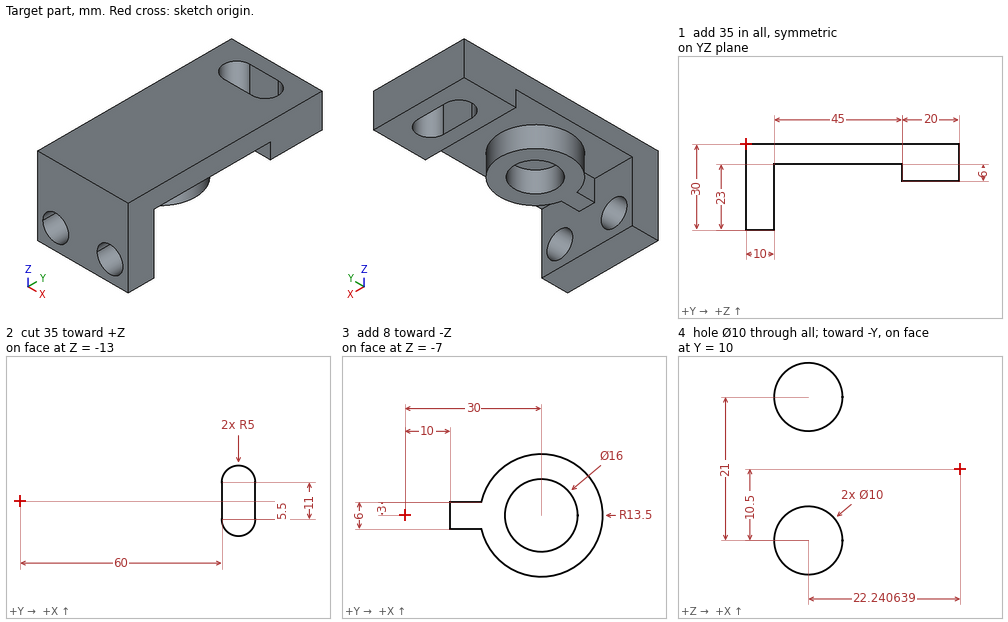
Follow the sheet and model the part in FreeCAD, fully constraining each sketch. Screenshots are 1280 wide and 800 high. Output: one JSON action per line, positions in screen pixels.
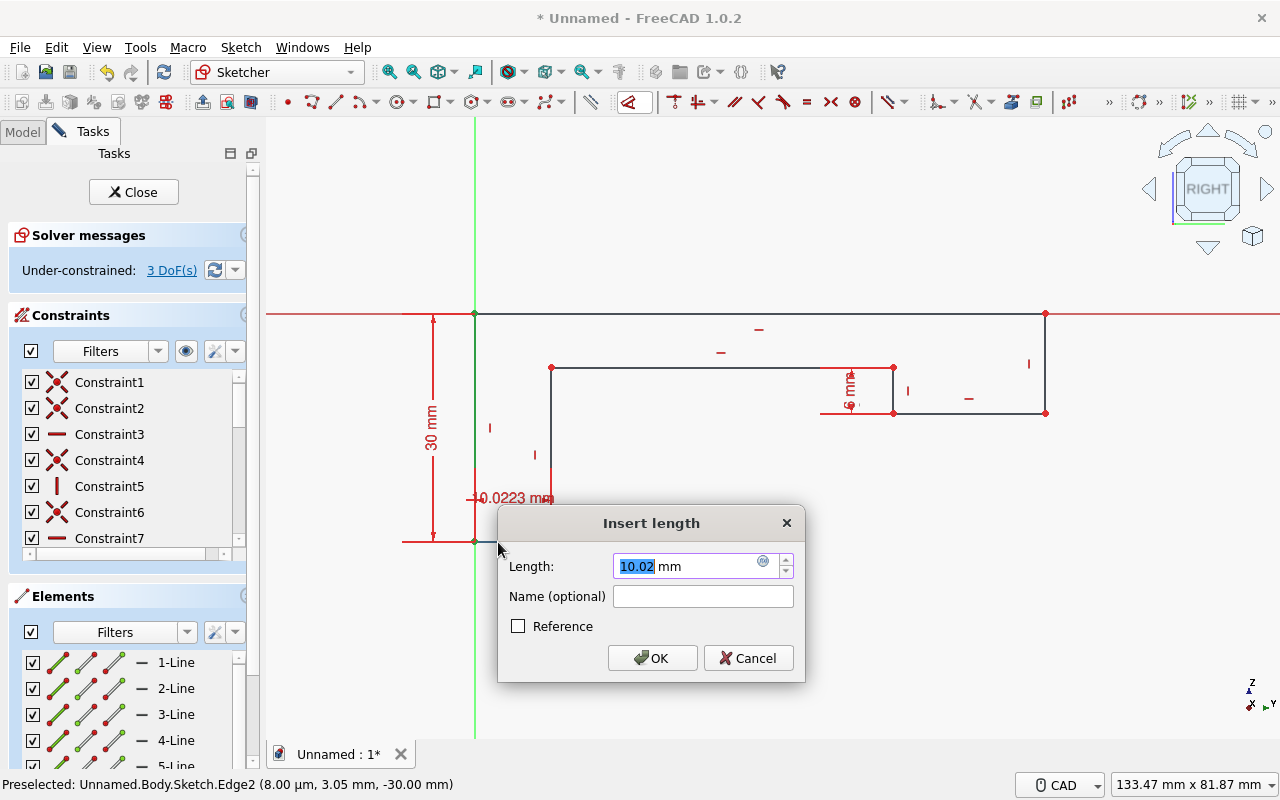
{"action": "type", "text": "10"}
{"action": "key", "text": "Return"}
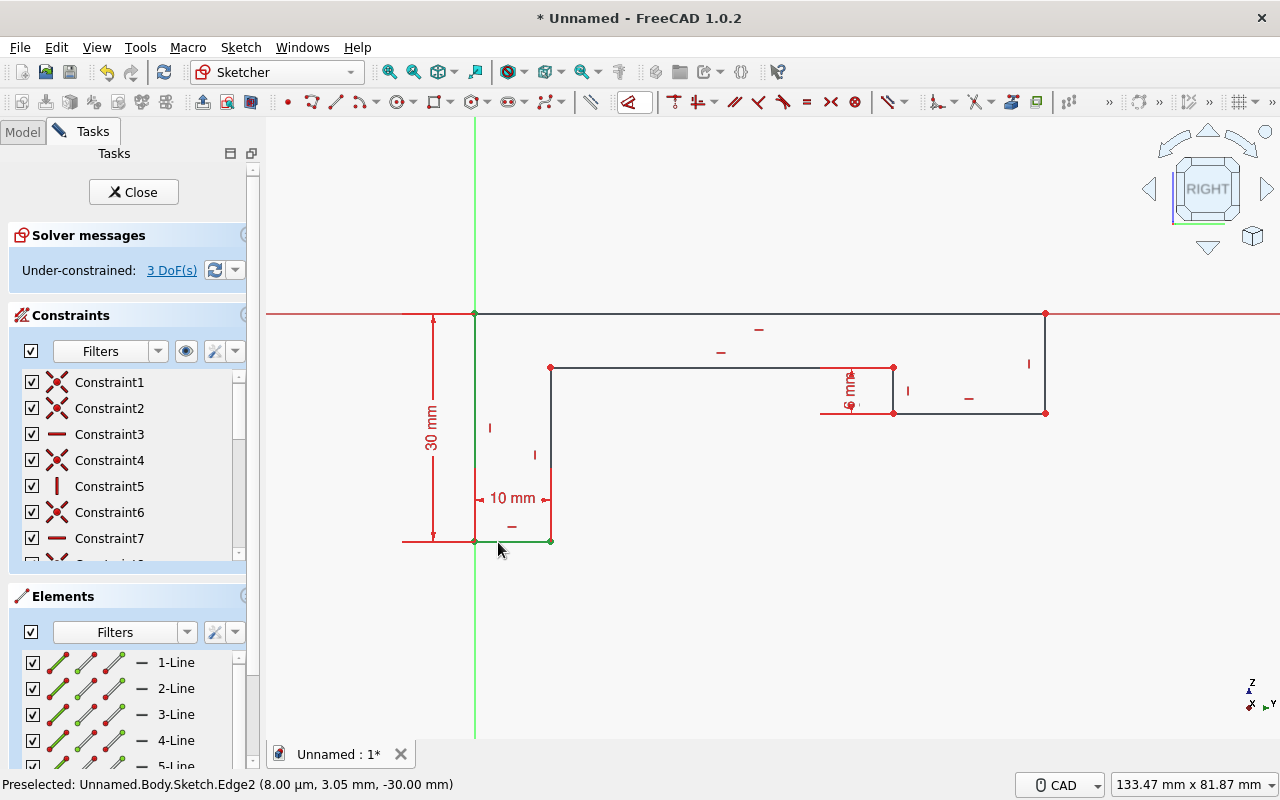
{"action": "left_click", "coordinate": [551, 490]}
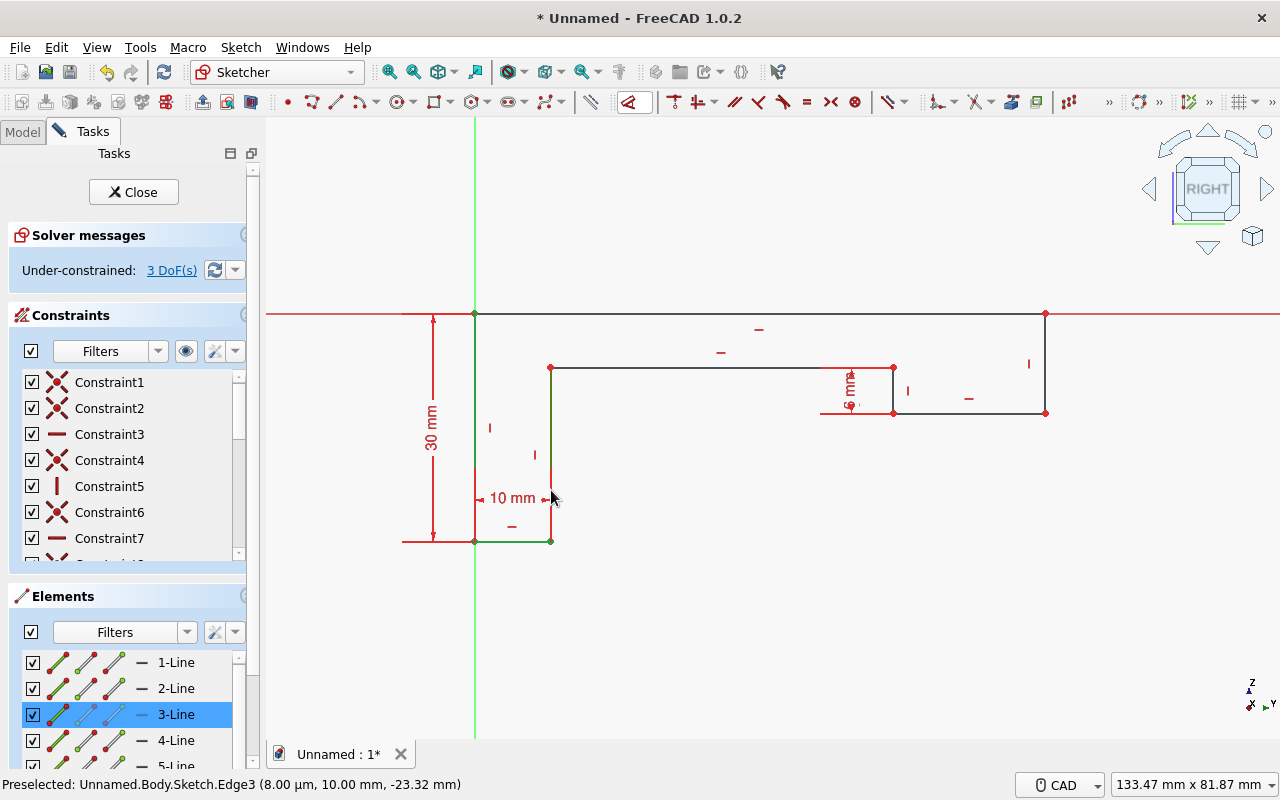
{"action": "key", "text": "i"}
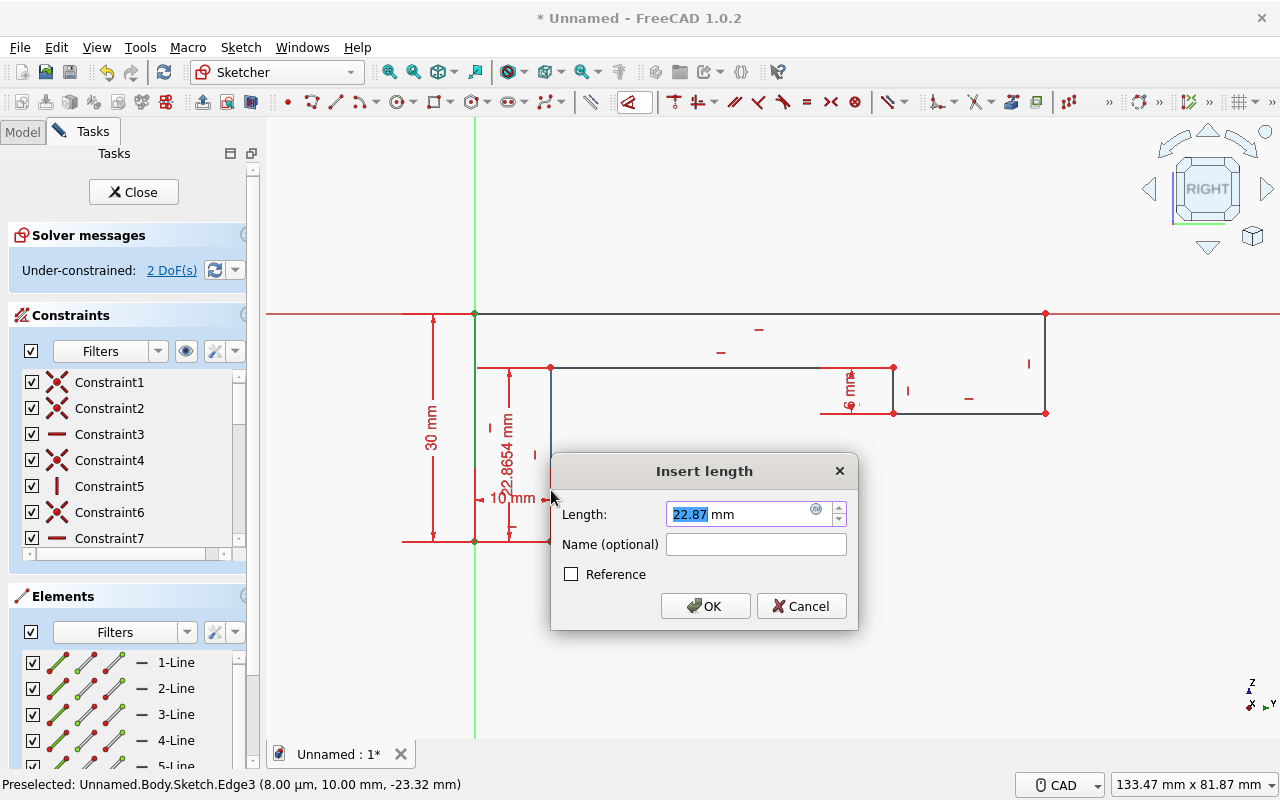
{"action": "type", "text": "23"}
{"action": "key", "text": "Return"}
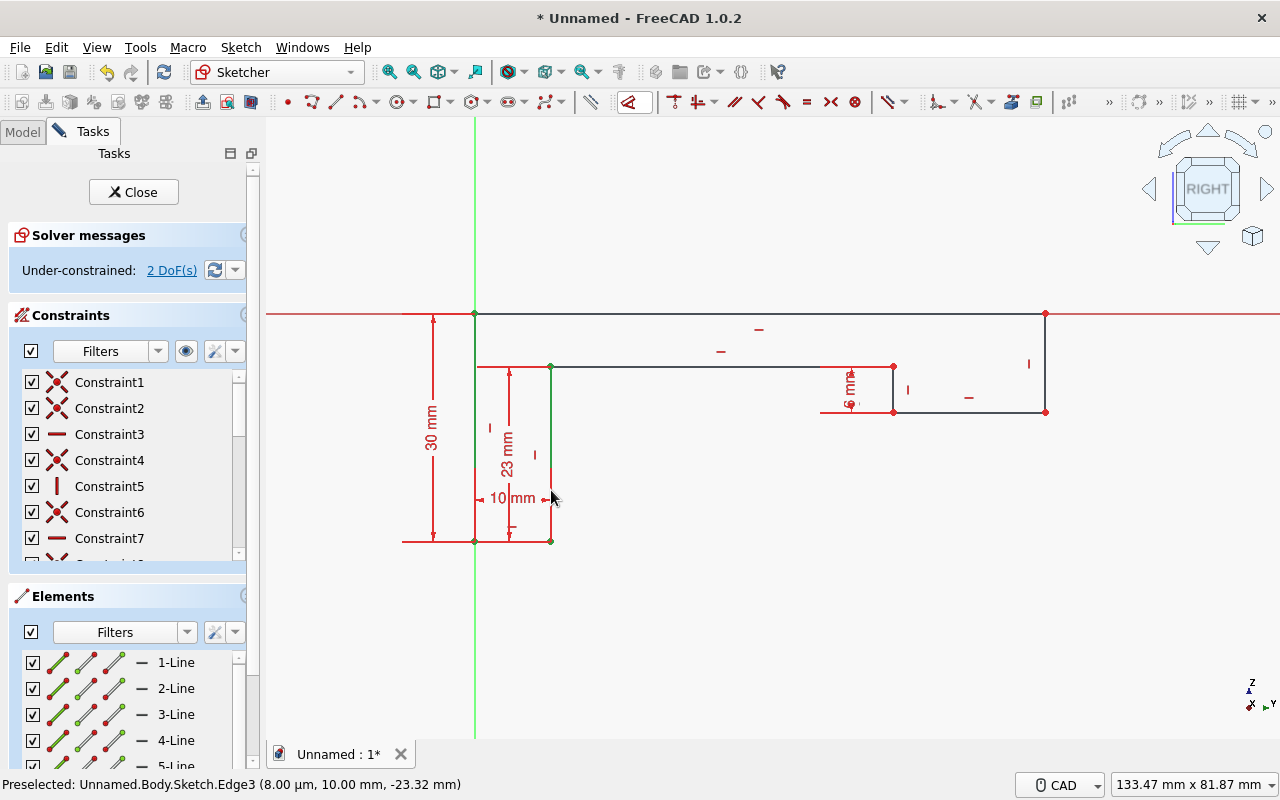
{"action": "left_click", "coordinate": [653, 367]}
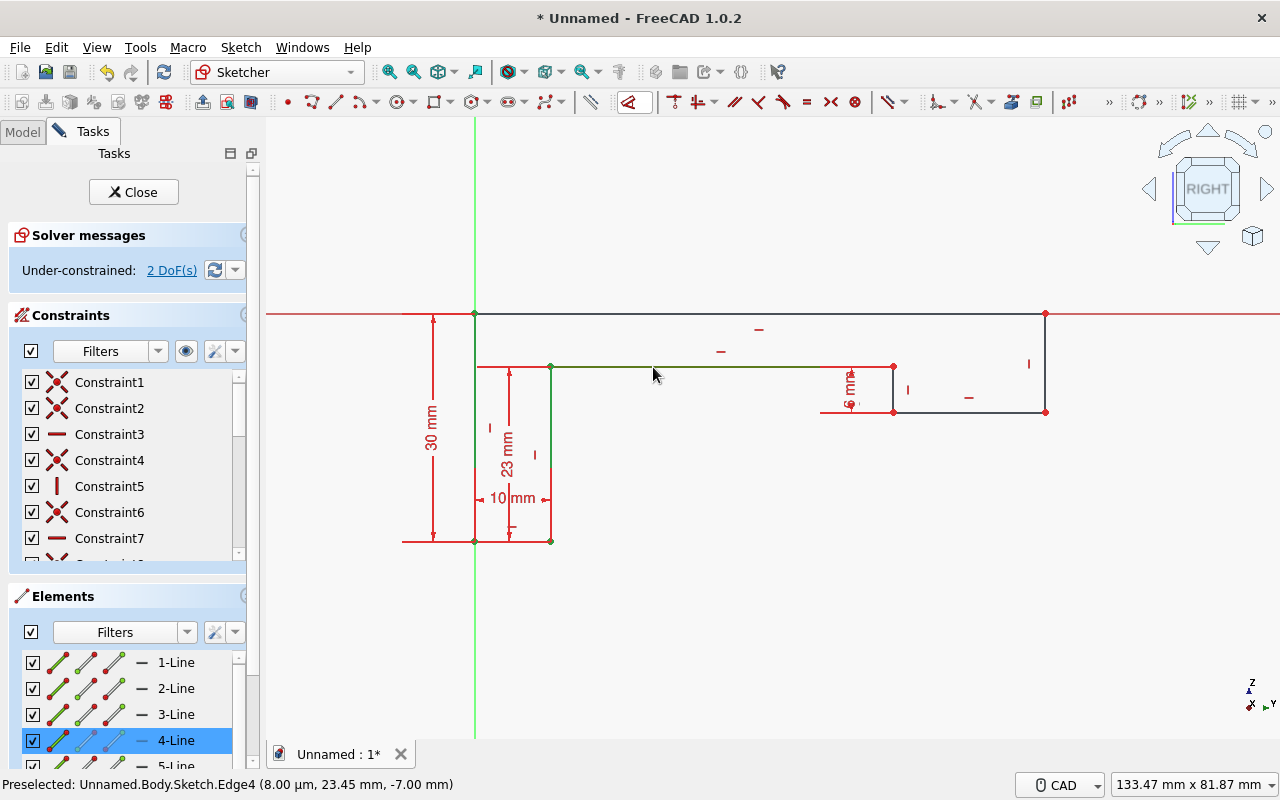
{"action": "left_click", "coordinate": [646, 102]}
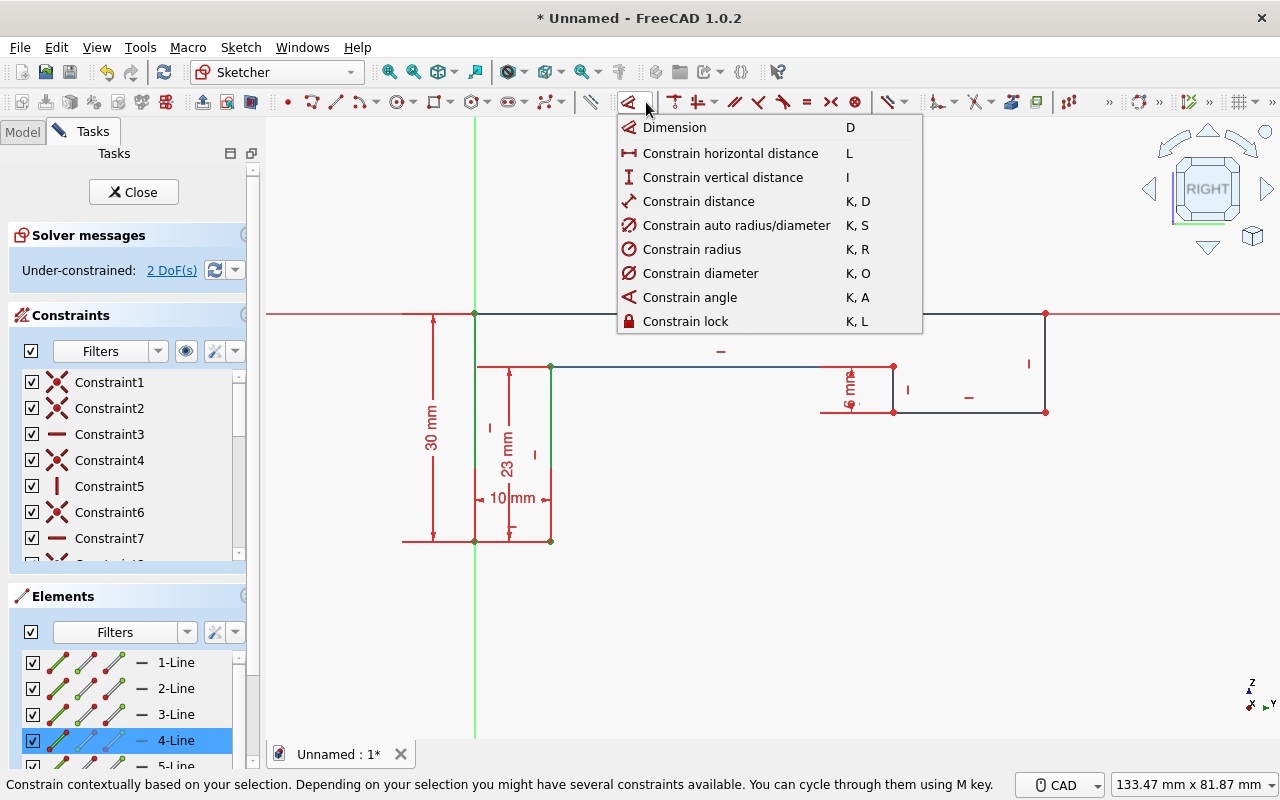
{"action": "left_click", "coordinate": [770, 153]}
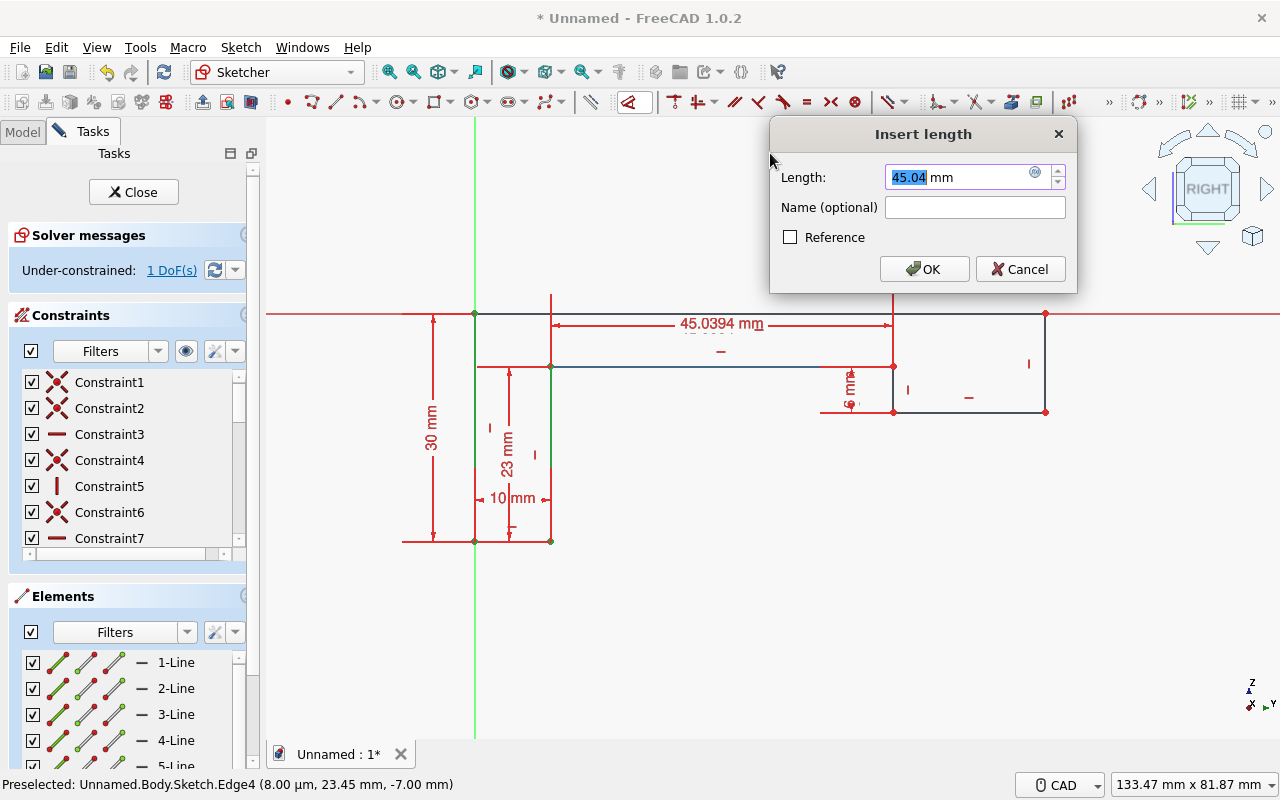
{"action": "type", "text": "45"}
{"action": "key", "text": "Return"}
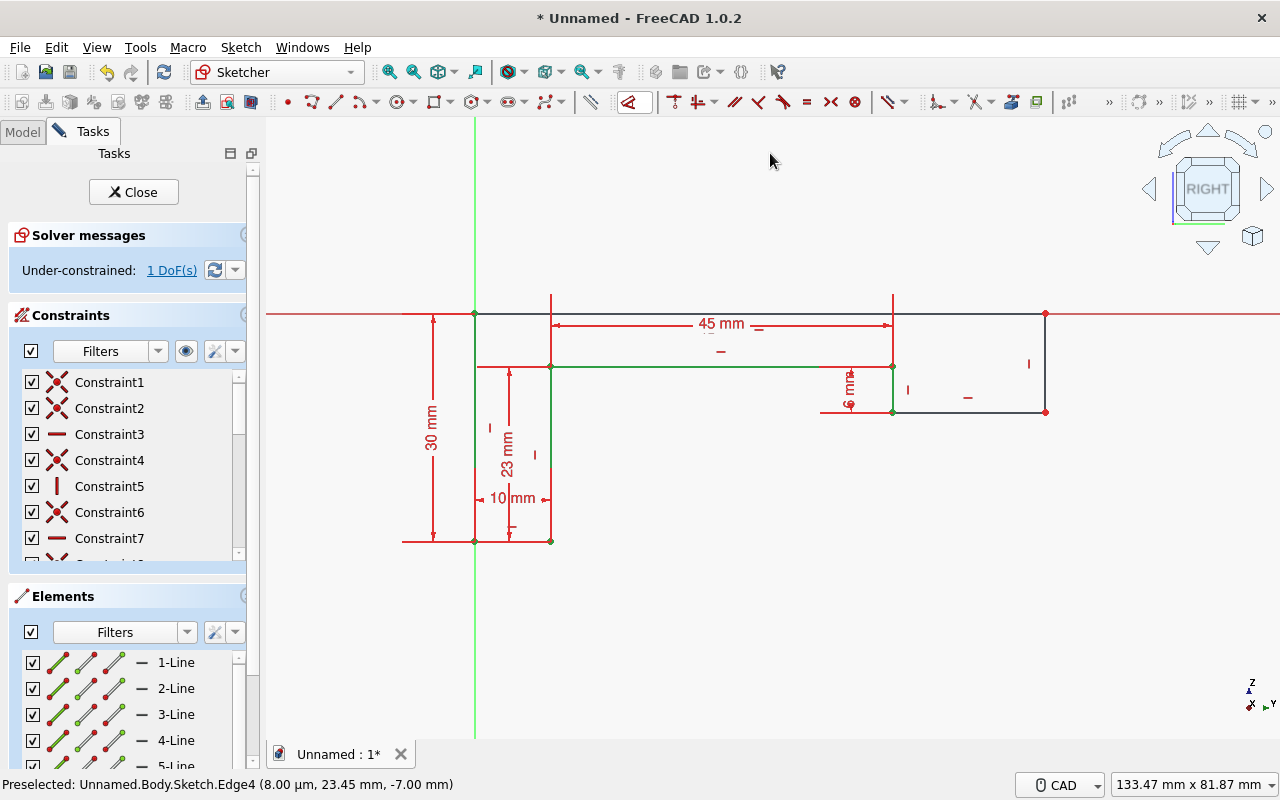
{"action": "left_click", "coordinate": [938, 413]}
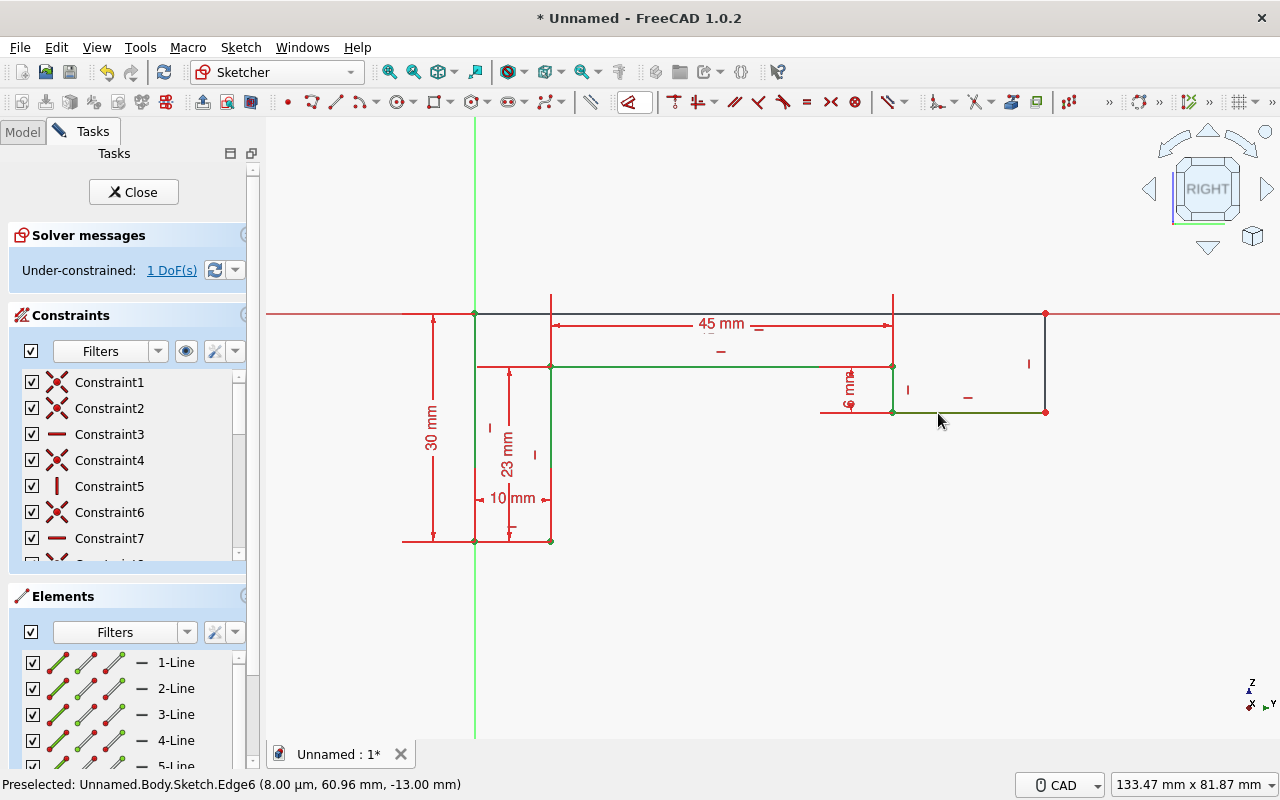
{"action": "left_click", "coordinate": [646, 102]}